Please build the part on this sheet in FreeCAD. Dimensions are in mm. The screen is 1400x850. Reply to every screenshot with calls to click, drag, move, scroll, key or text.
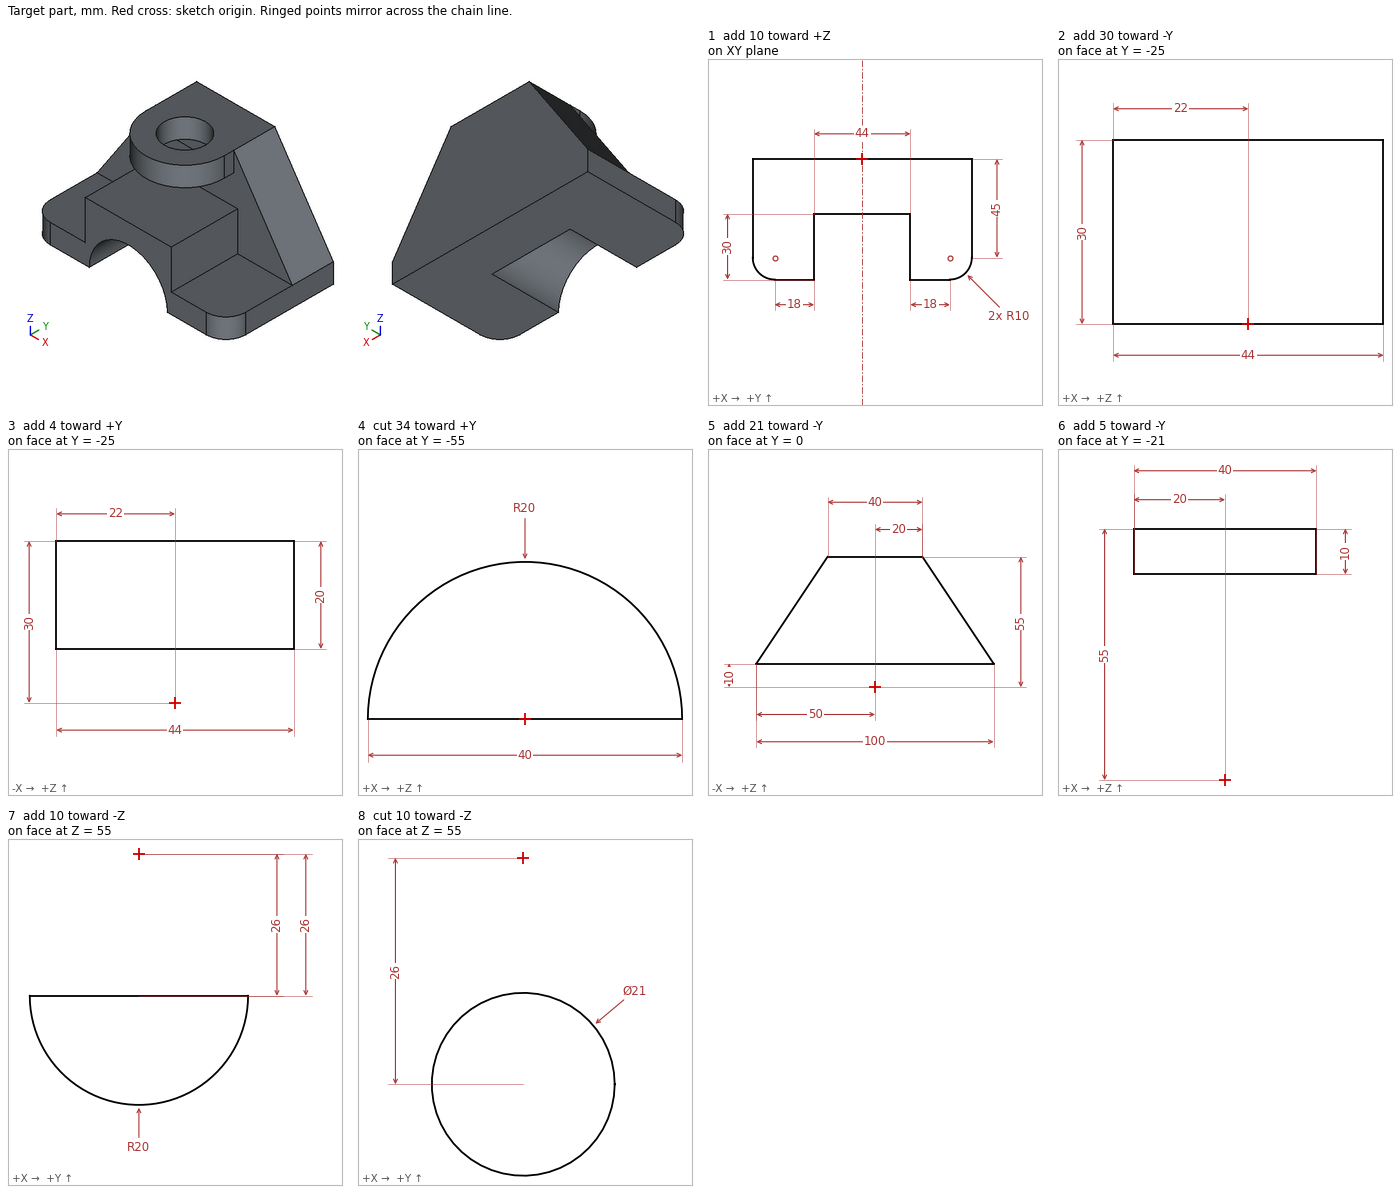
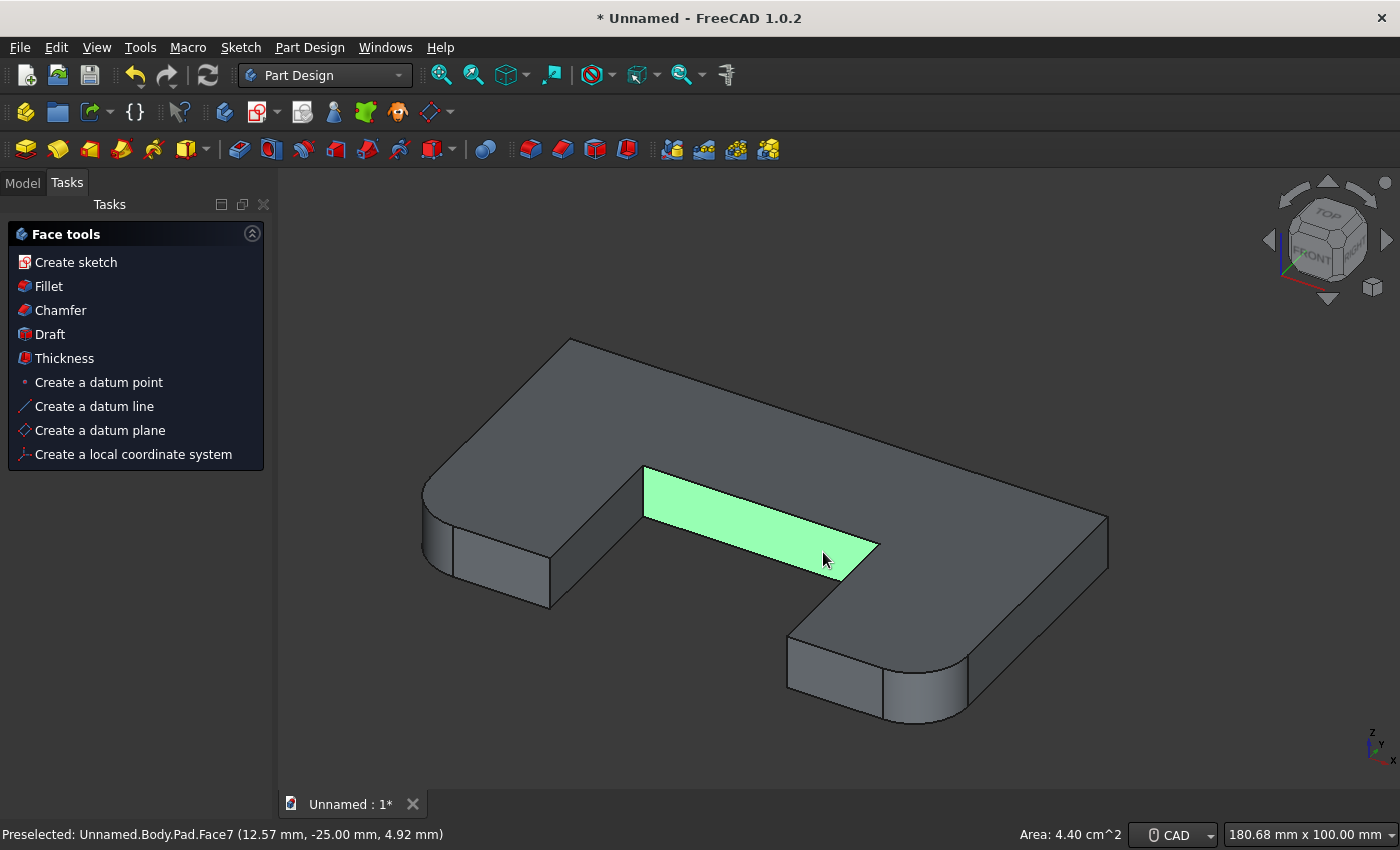
click(258, 112)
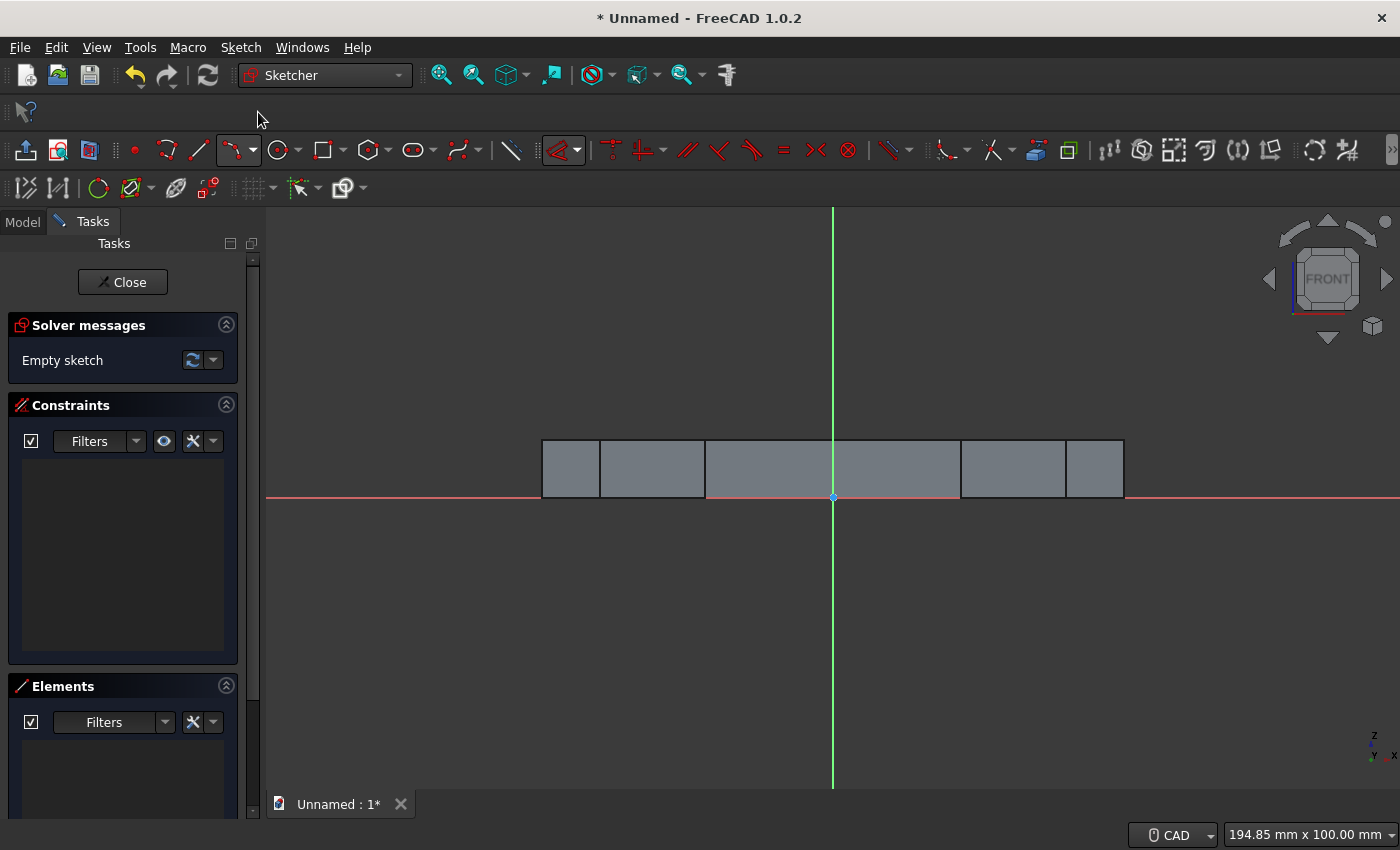
click(90, 150)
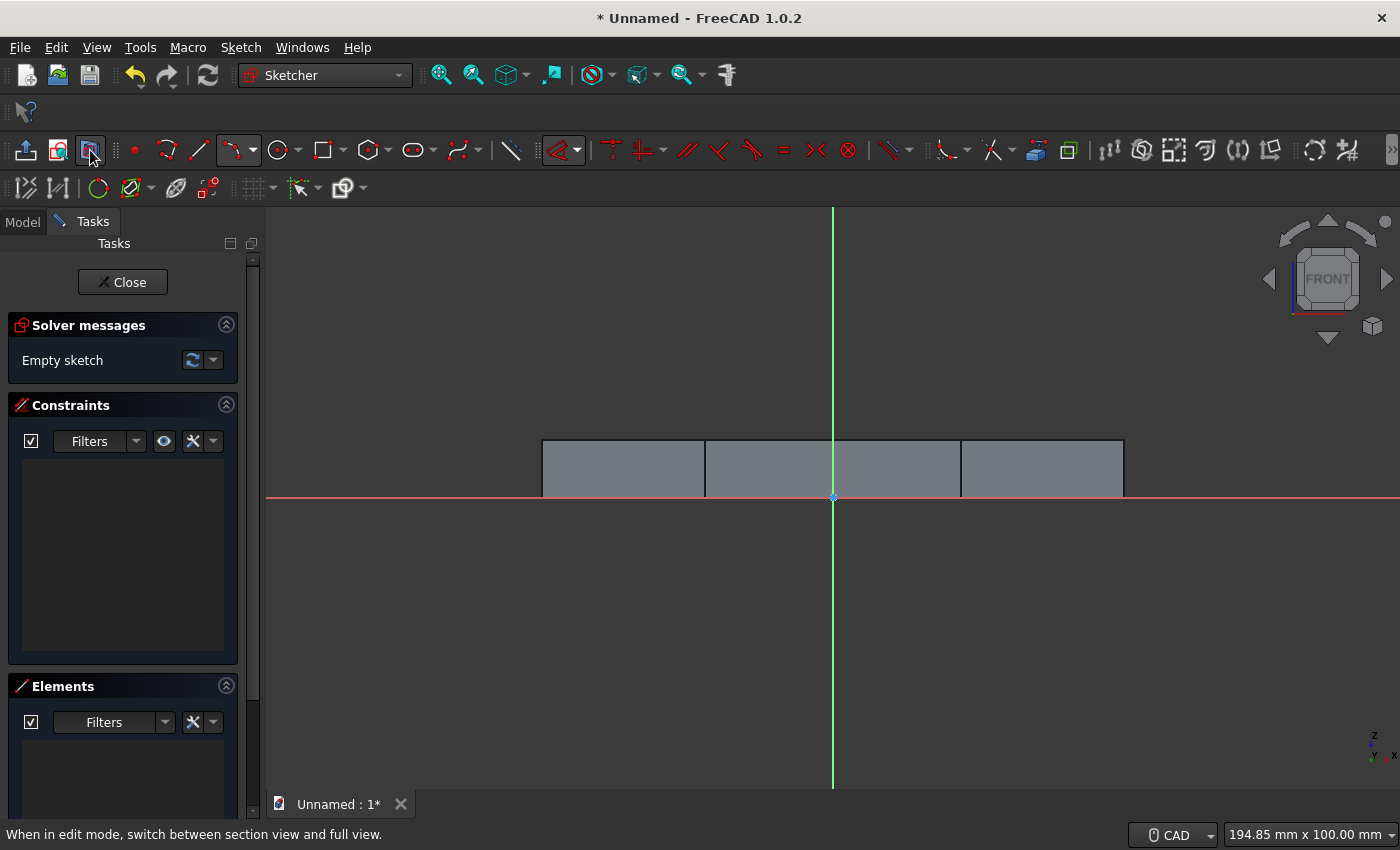
scroll(889, 339, up, 4)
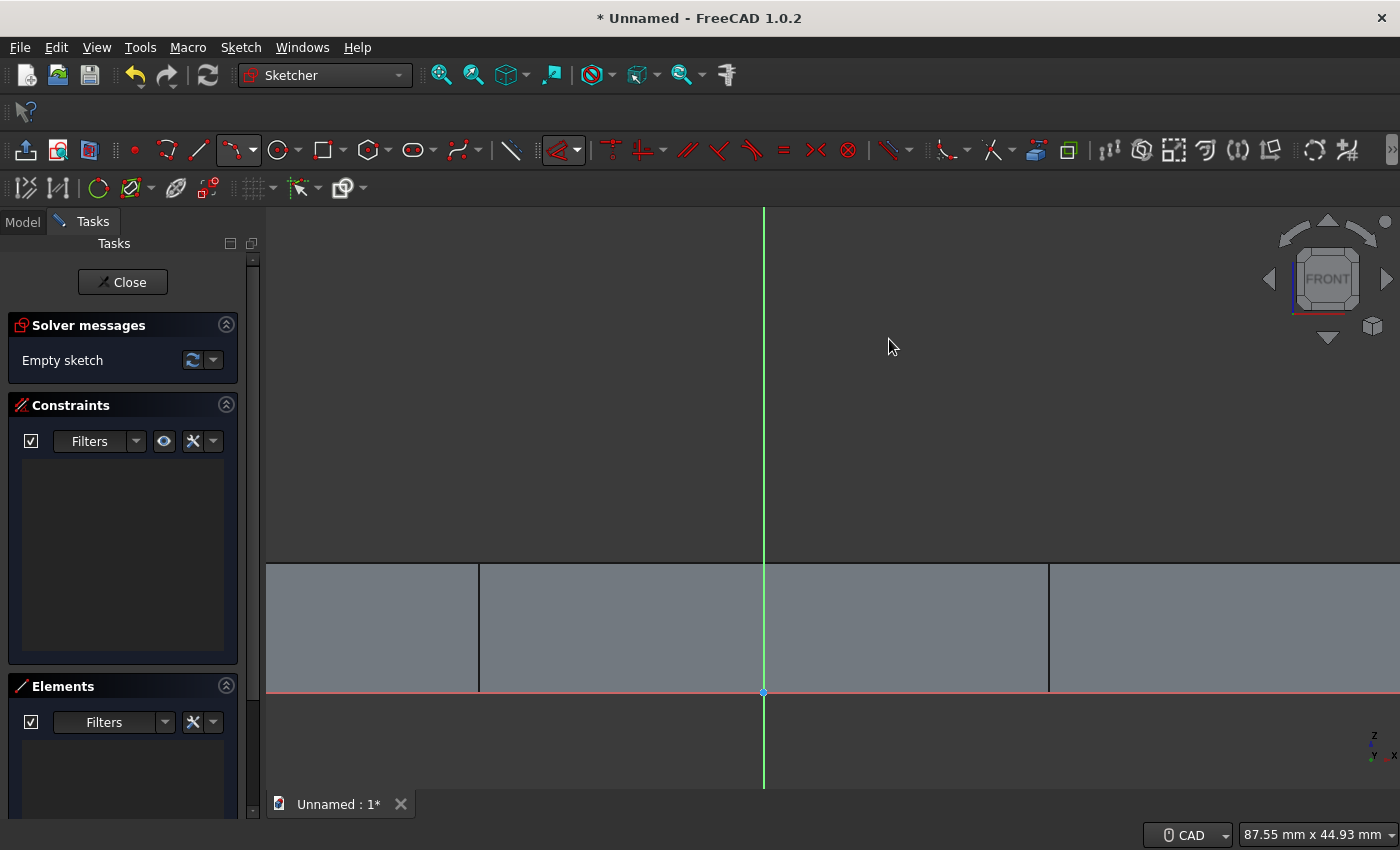
click(324, 150)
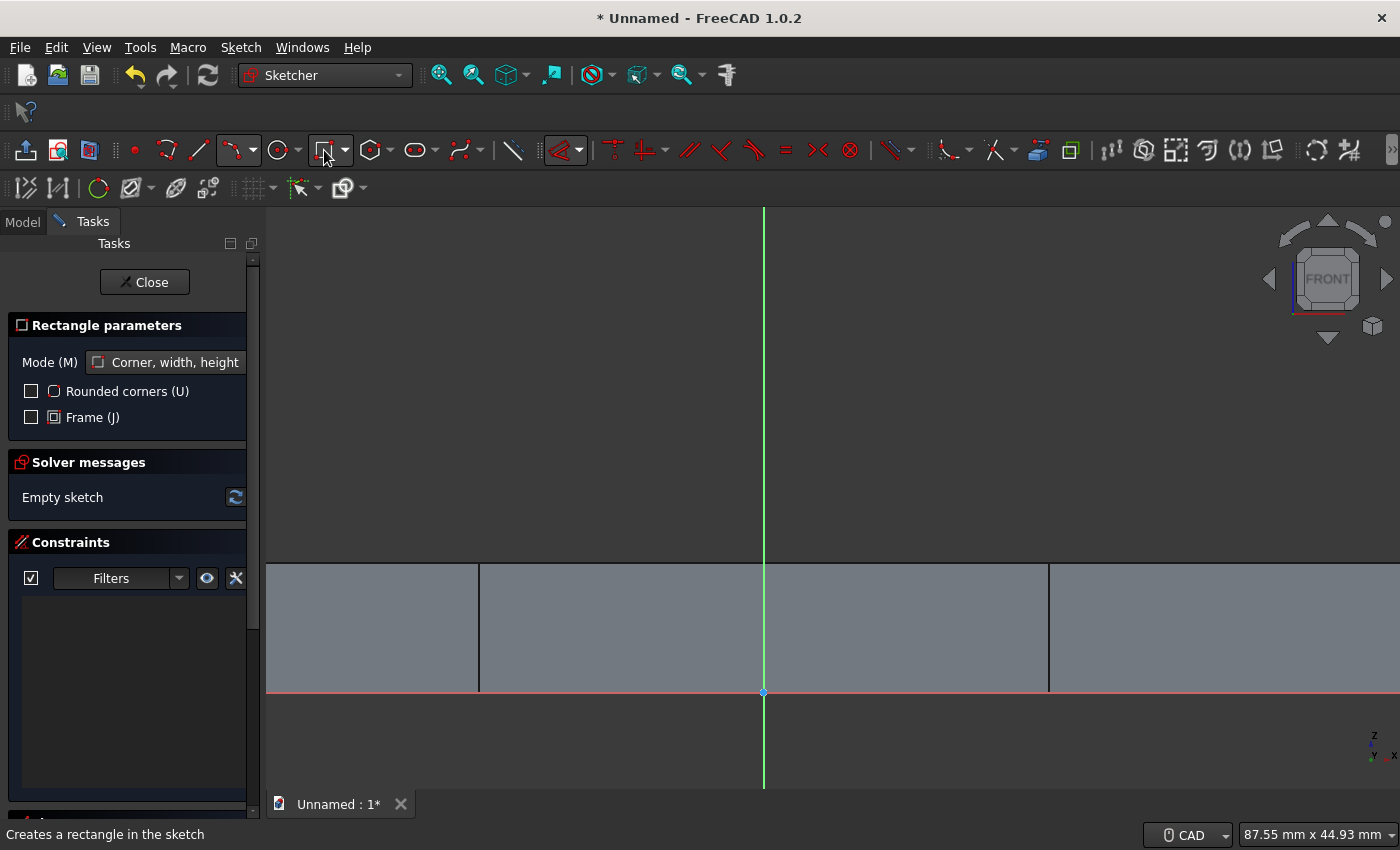
click(479, 304)
click(1049, 693)
key(Escape)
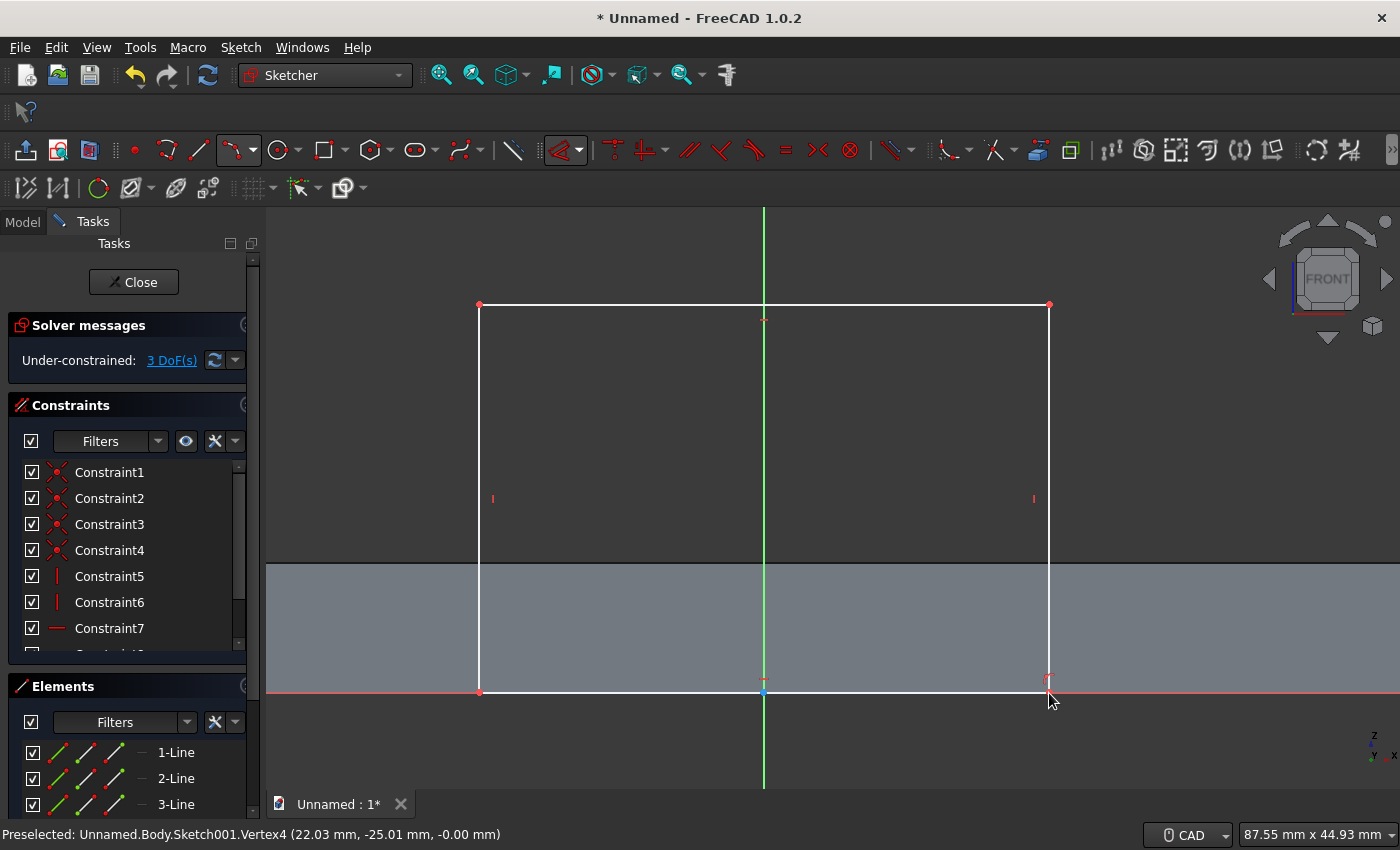
click(479, 421)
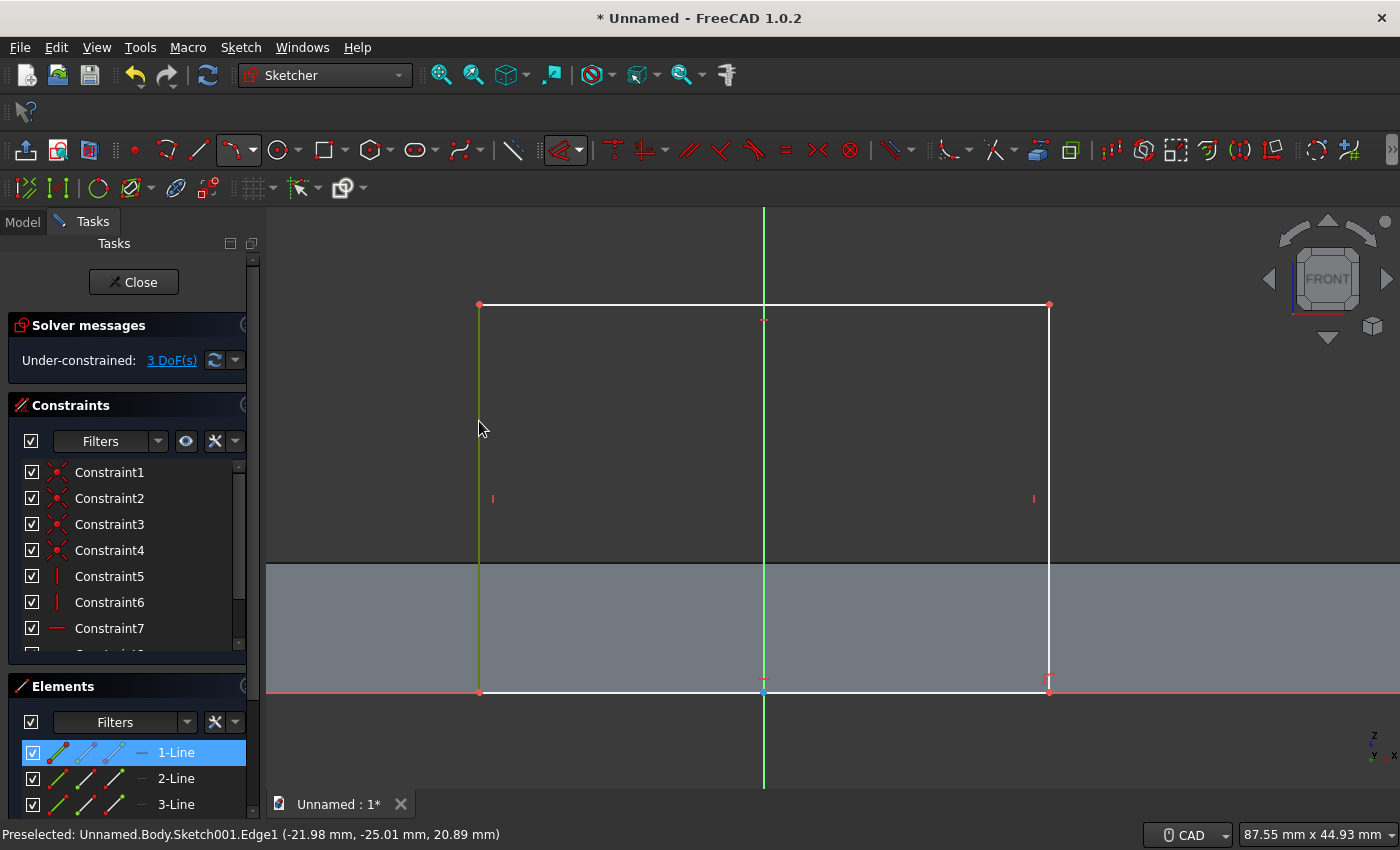
click(582, 150)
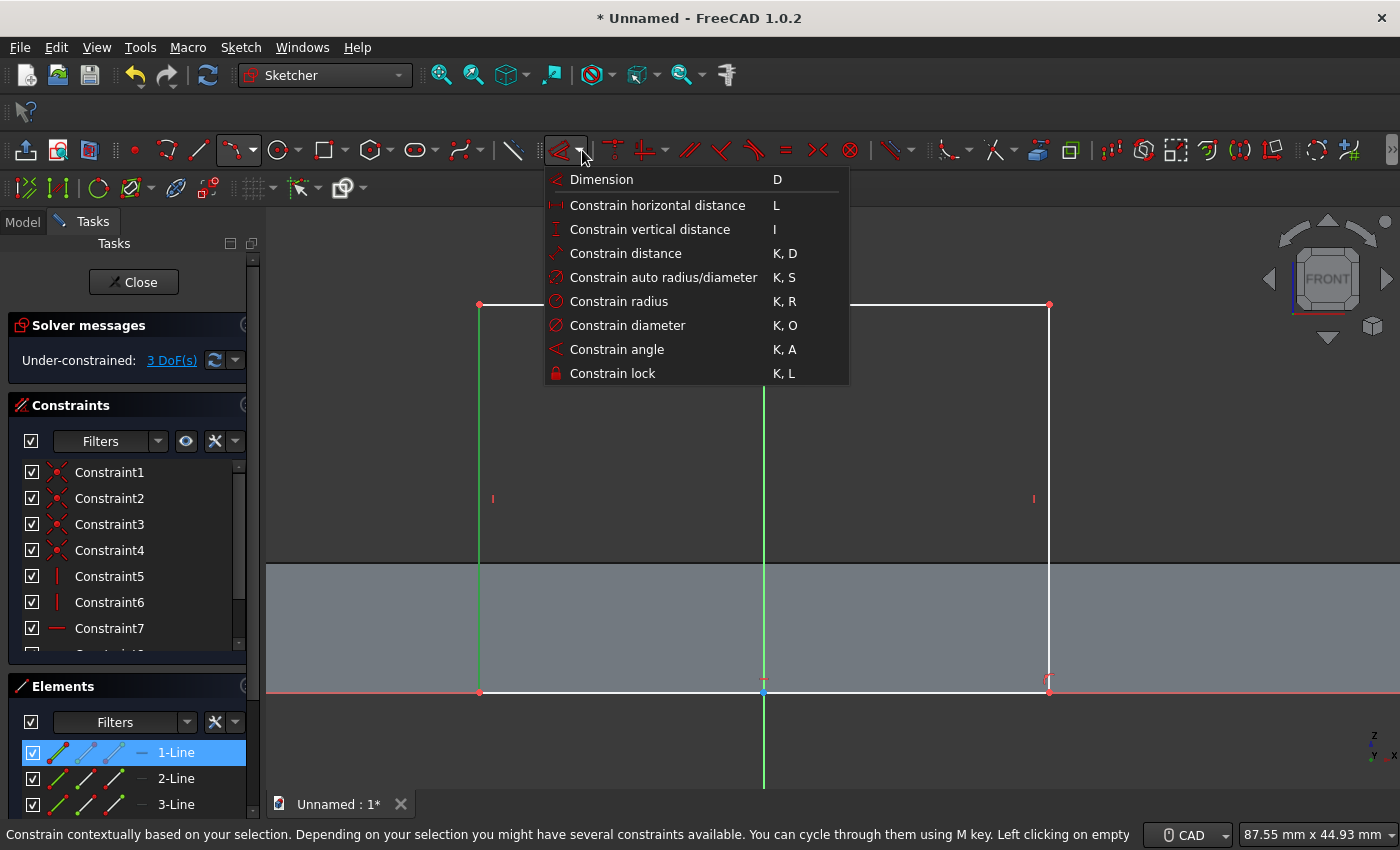
click(697, 229)